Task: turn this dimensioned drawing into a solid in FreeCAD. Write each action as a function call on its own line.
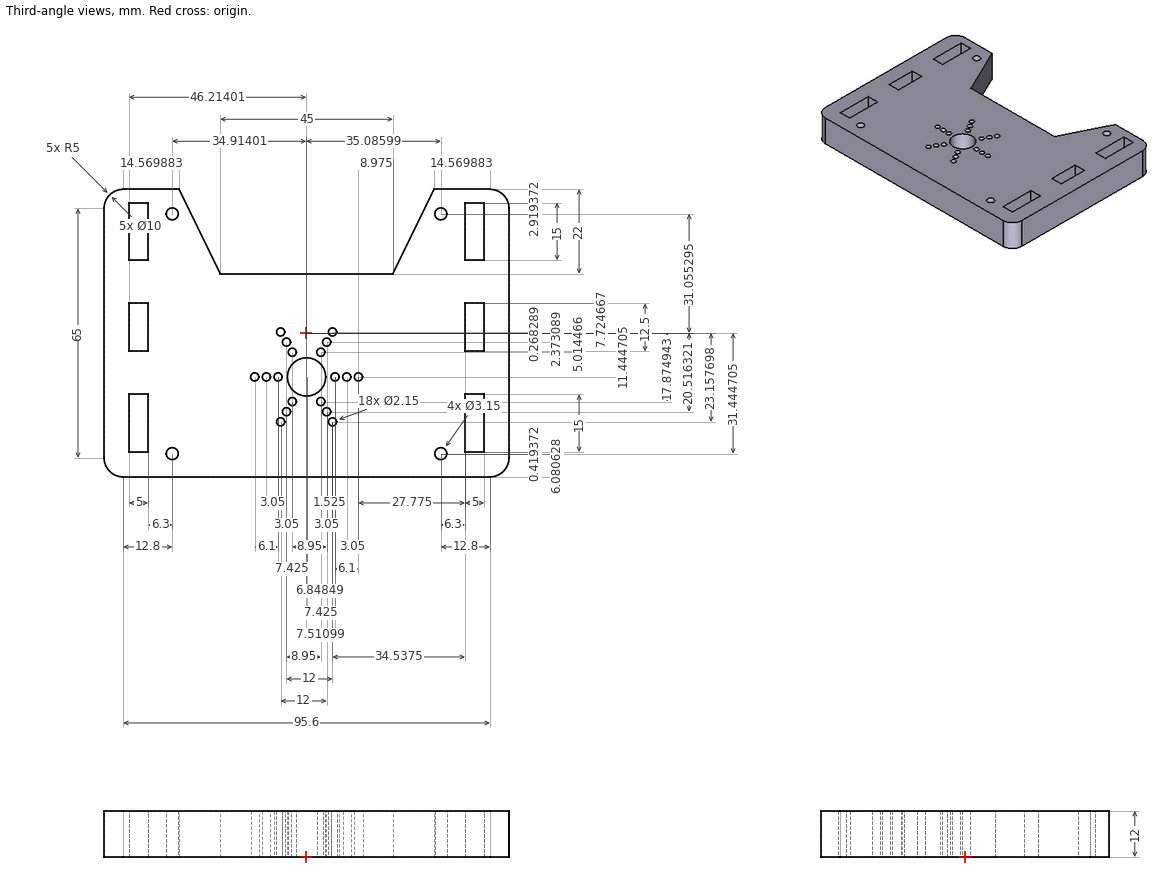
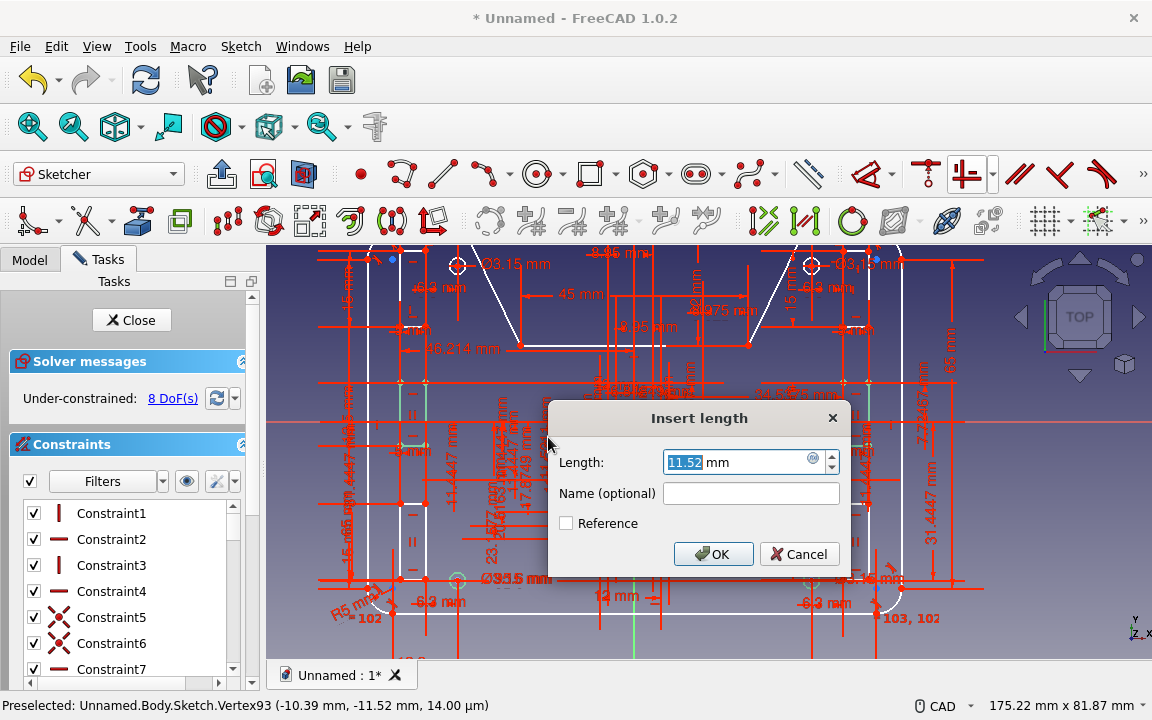
text(11.444705)
key(Return)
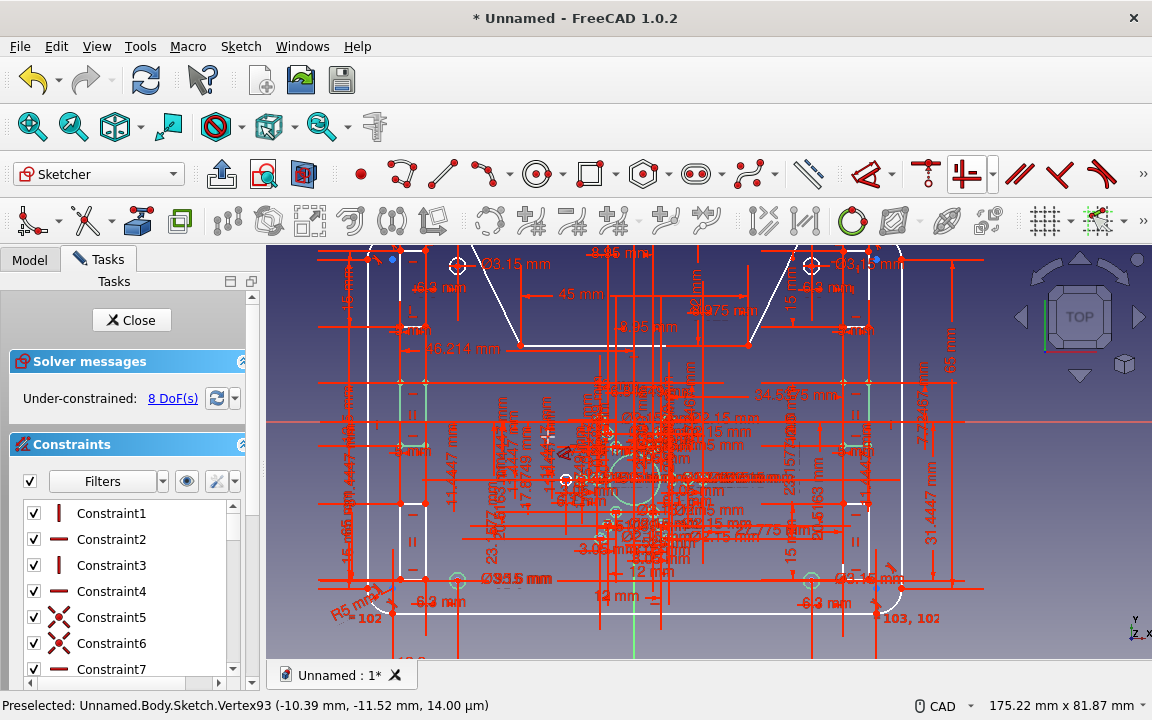
click(566, 480)
click(386, 437)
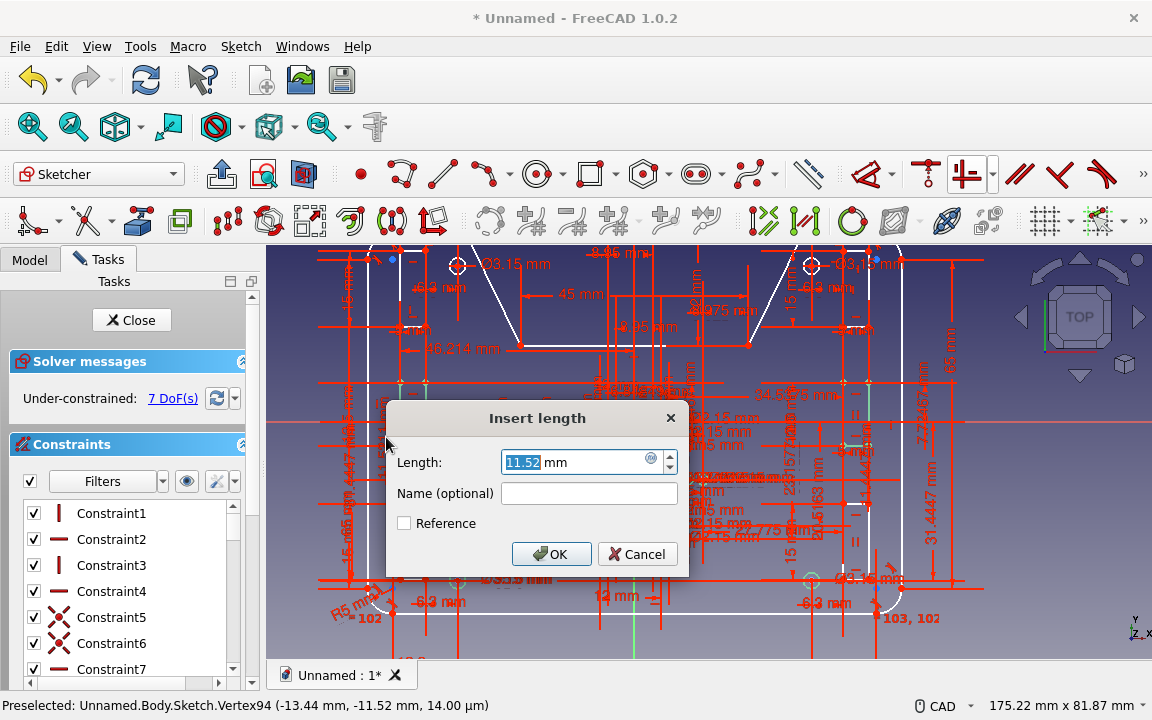
text(11.444705)
key(Return)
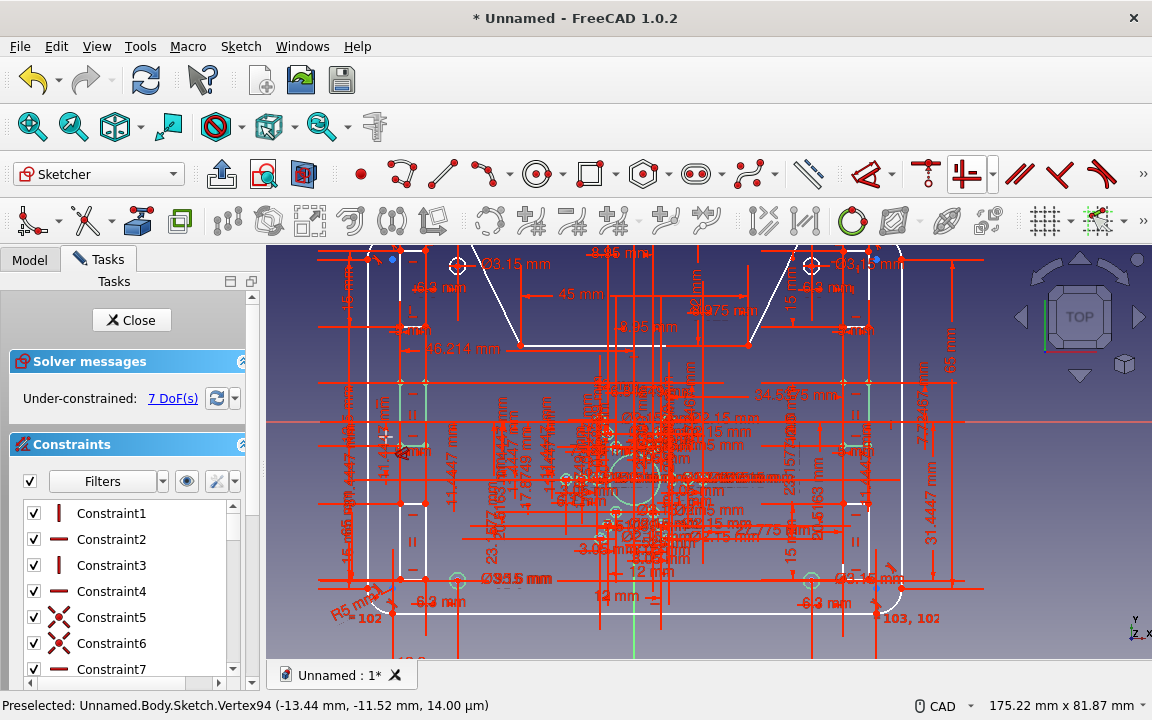
scroll(653, 513, down, 2)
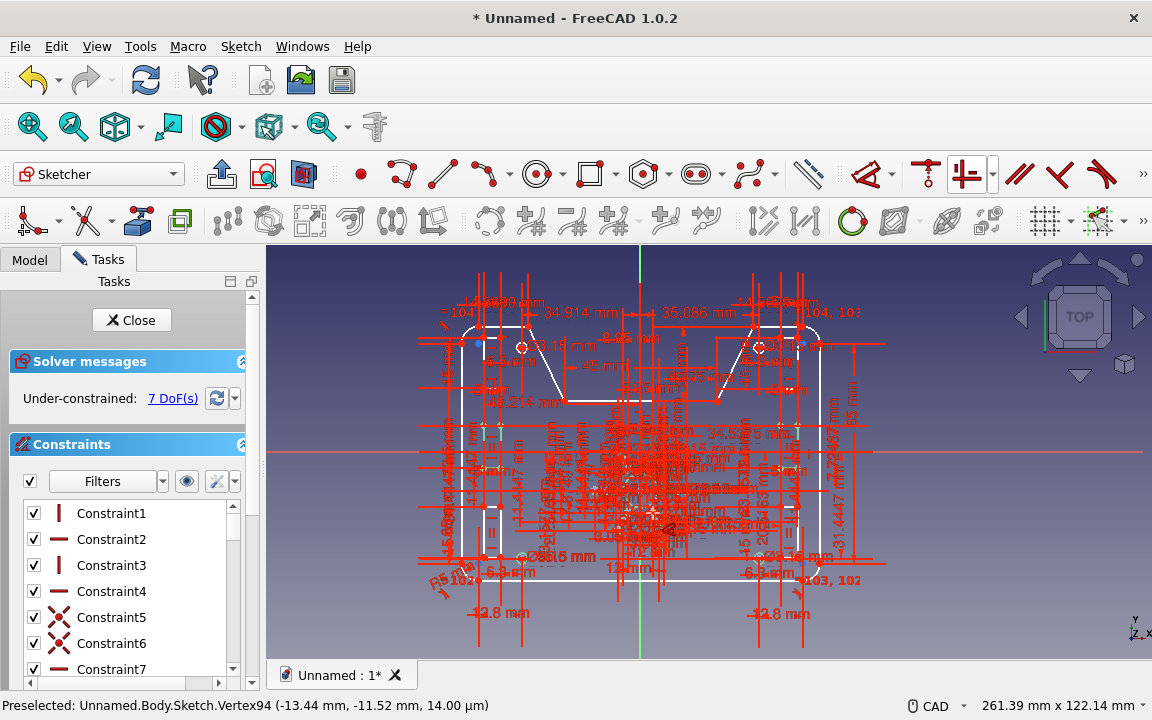
click(759, 348)
click(841, 376)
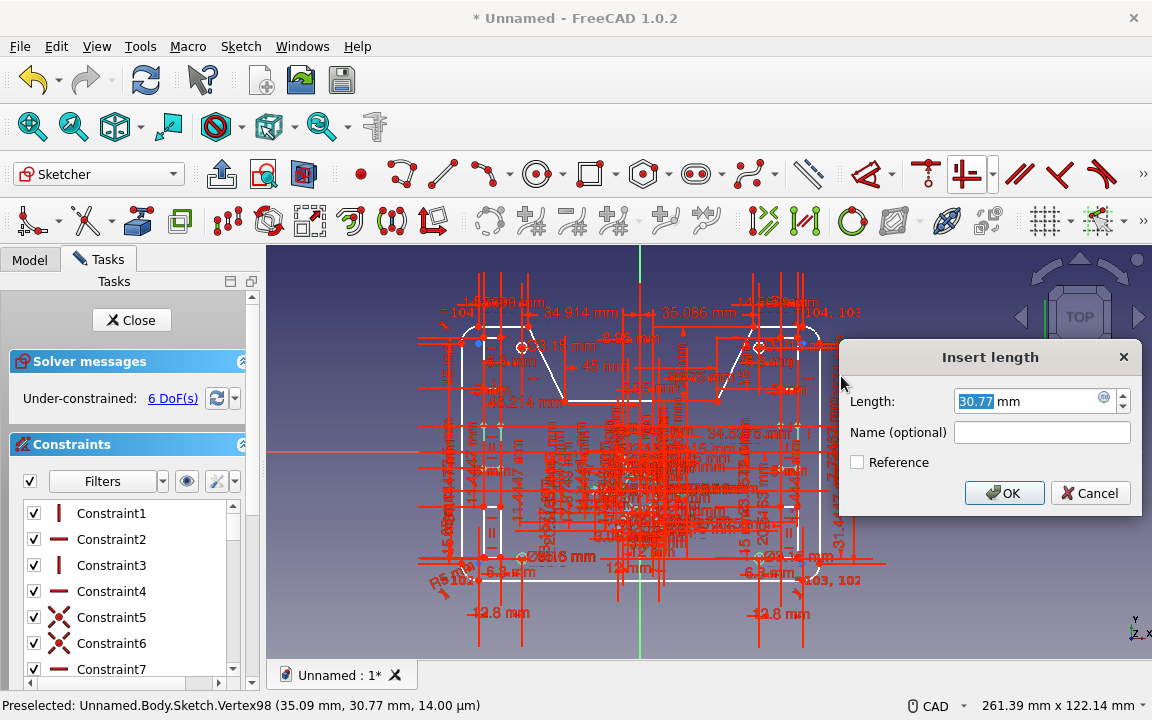
text(31.055295)
key(Return)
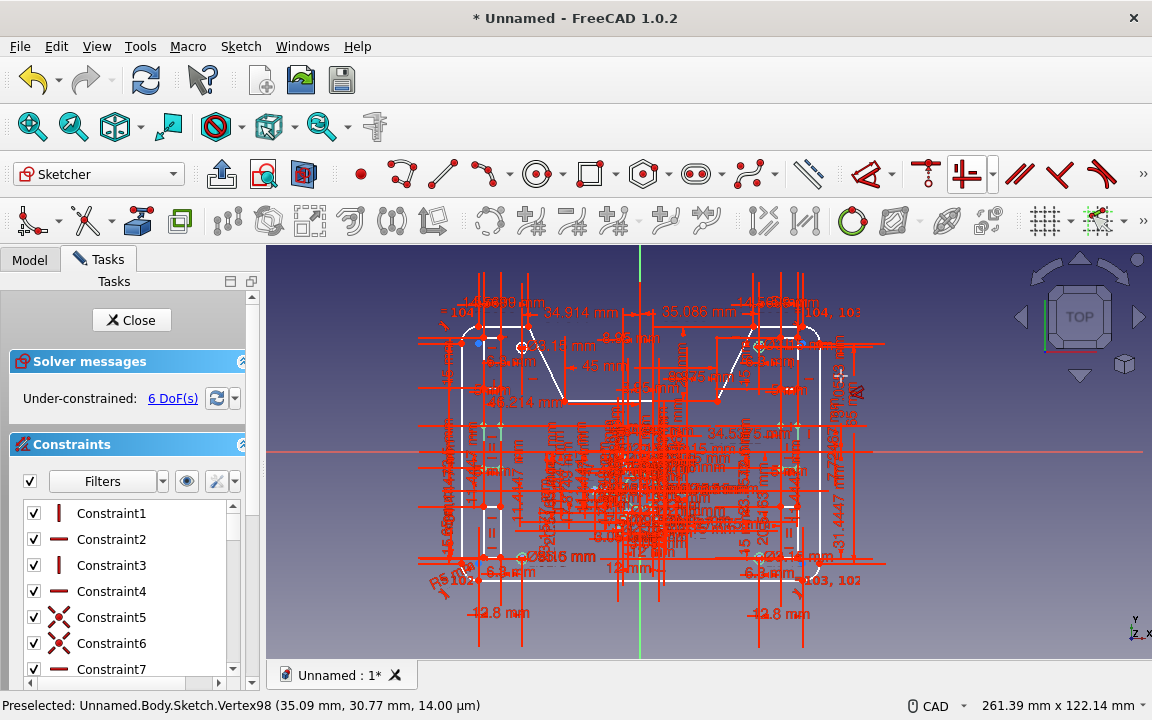
click(522, 348)
click(440, 400)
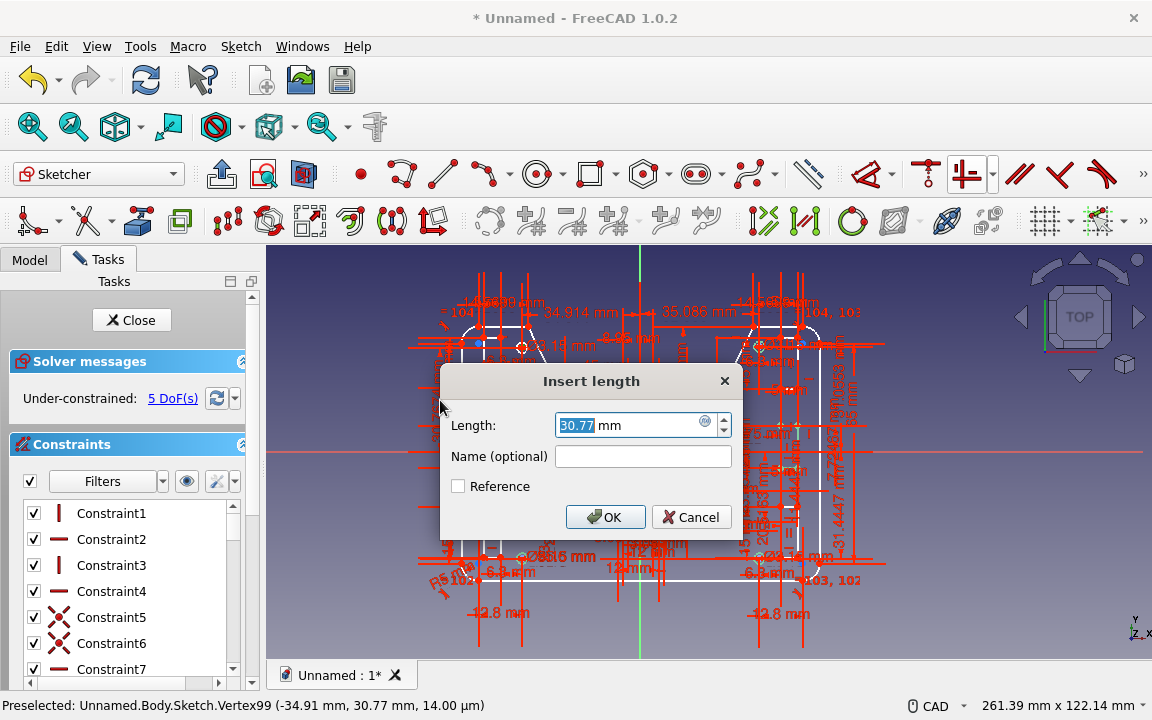
text(31.055295)
key(Return)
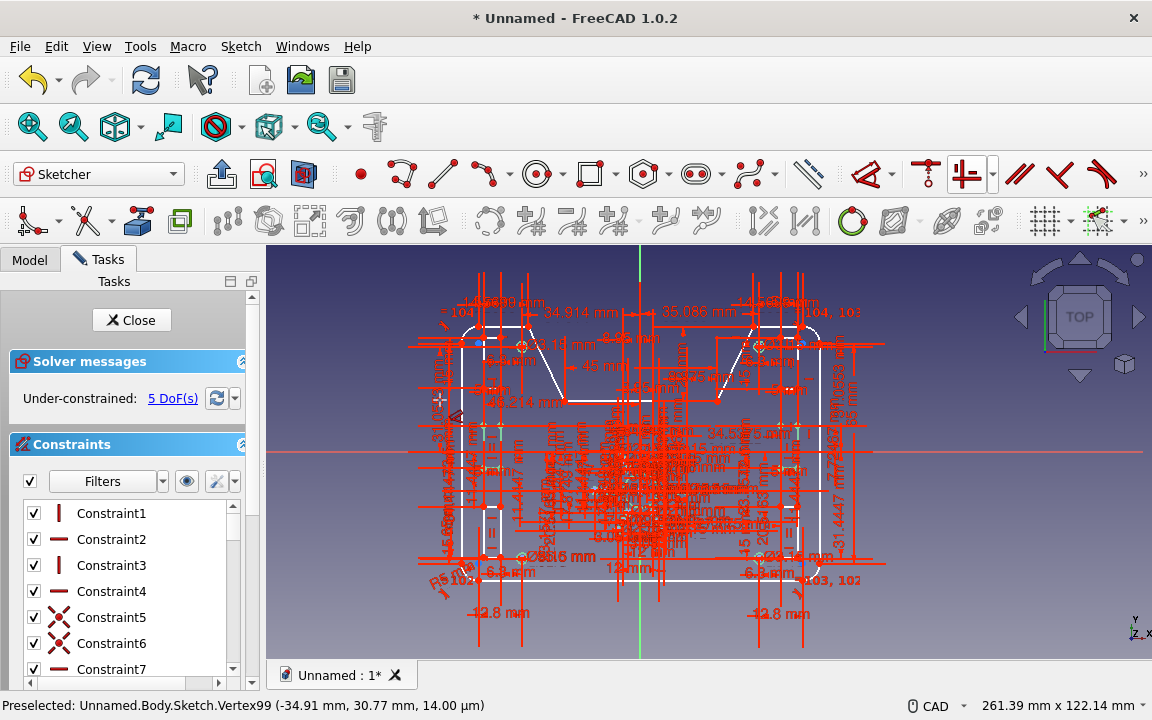
scroll(781, 558, up, 17)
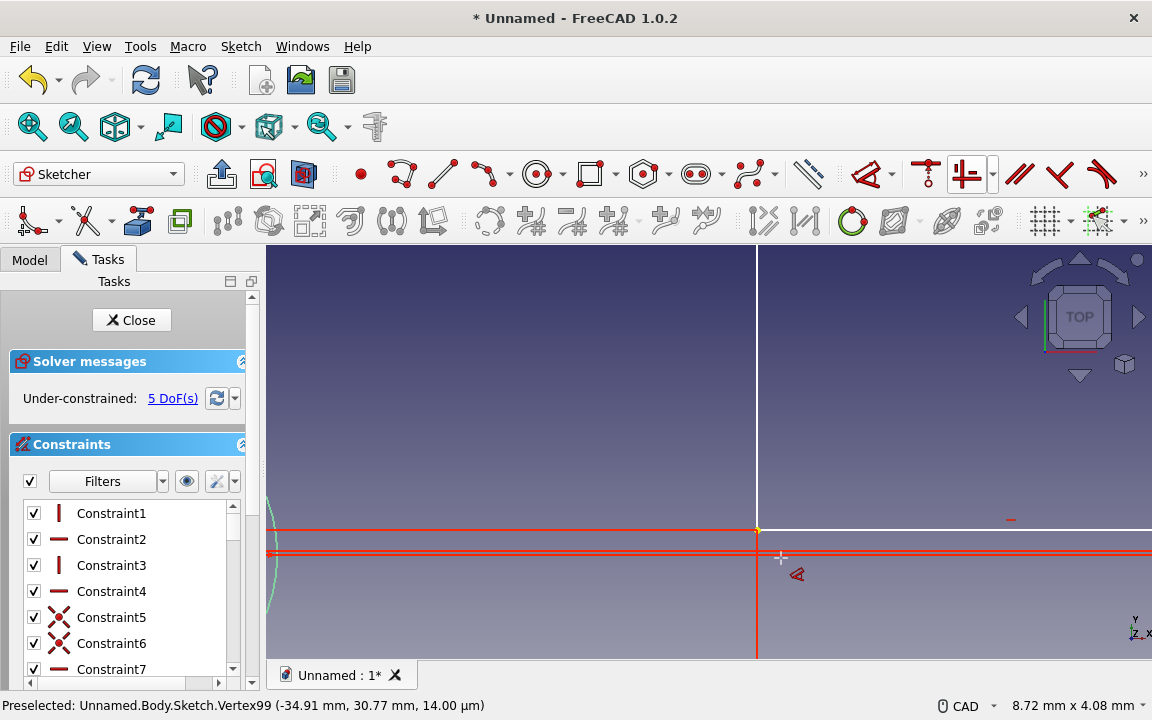
click(757, 530)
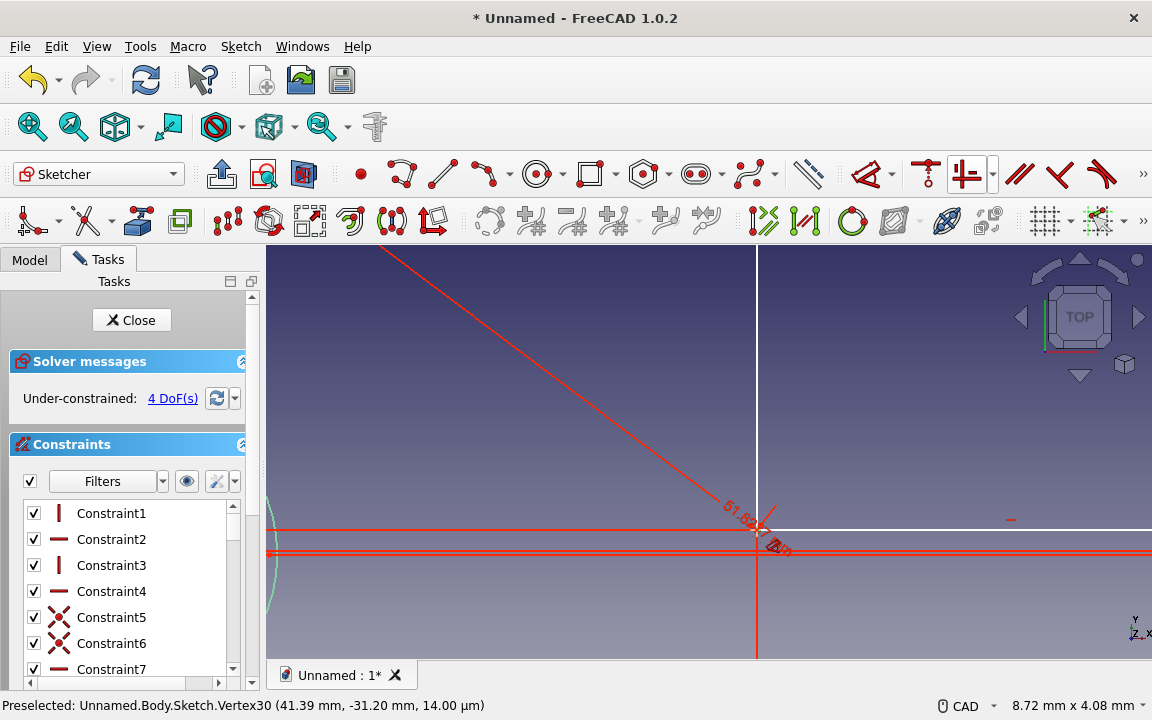
scroll(781, 559, down, 17)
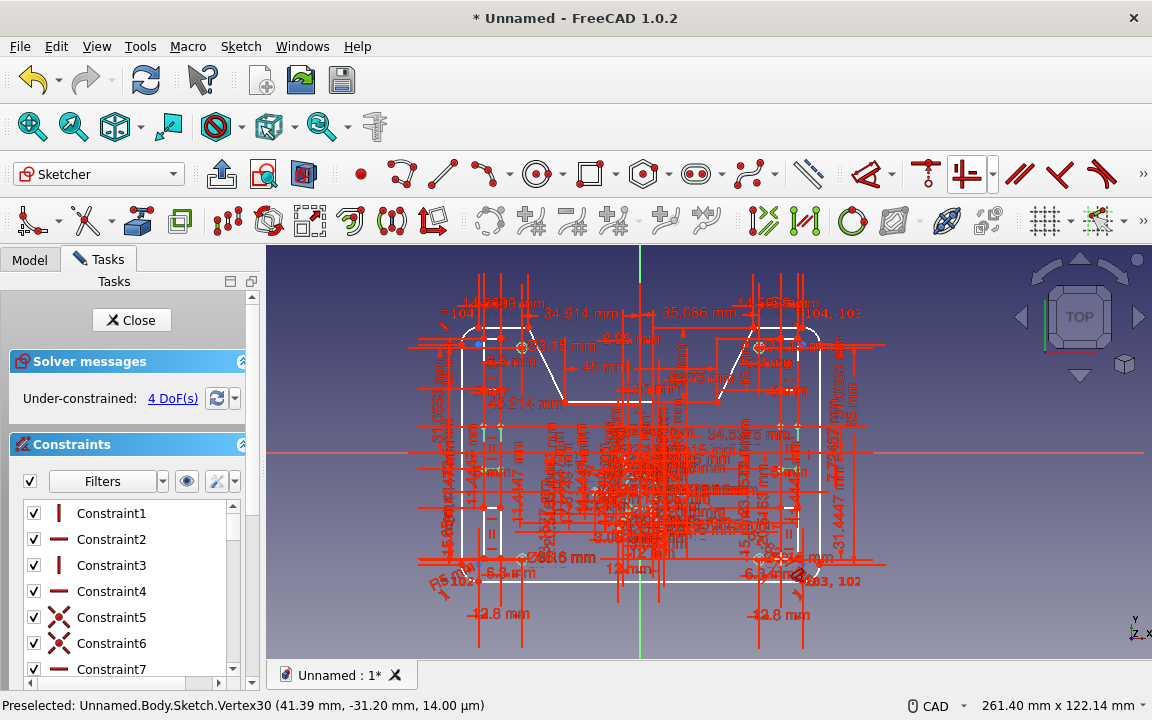
scroll(759, 560, up, 17)